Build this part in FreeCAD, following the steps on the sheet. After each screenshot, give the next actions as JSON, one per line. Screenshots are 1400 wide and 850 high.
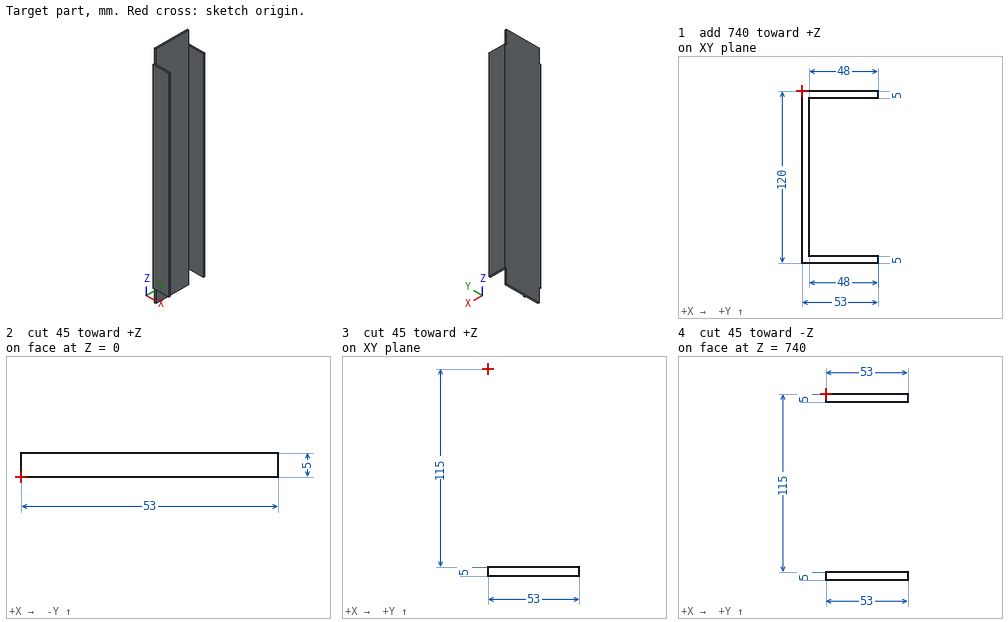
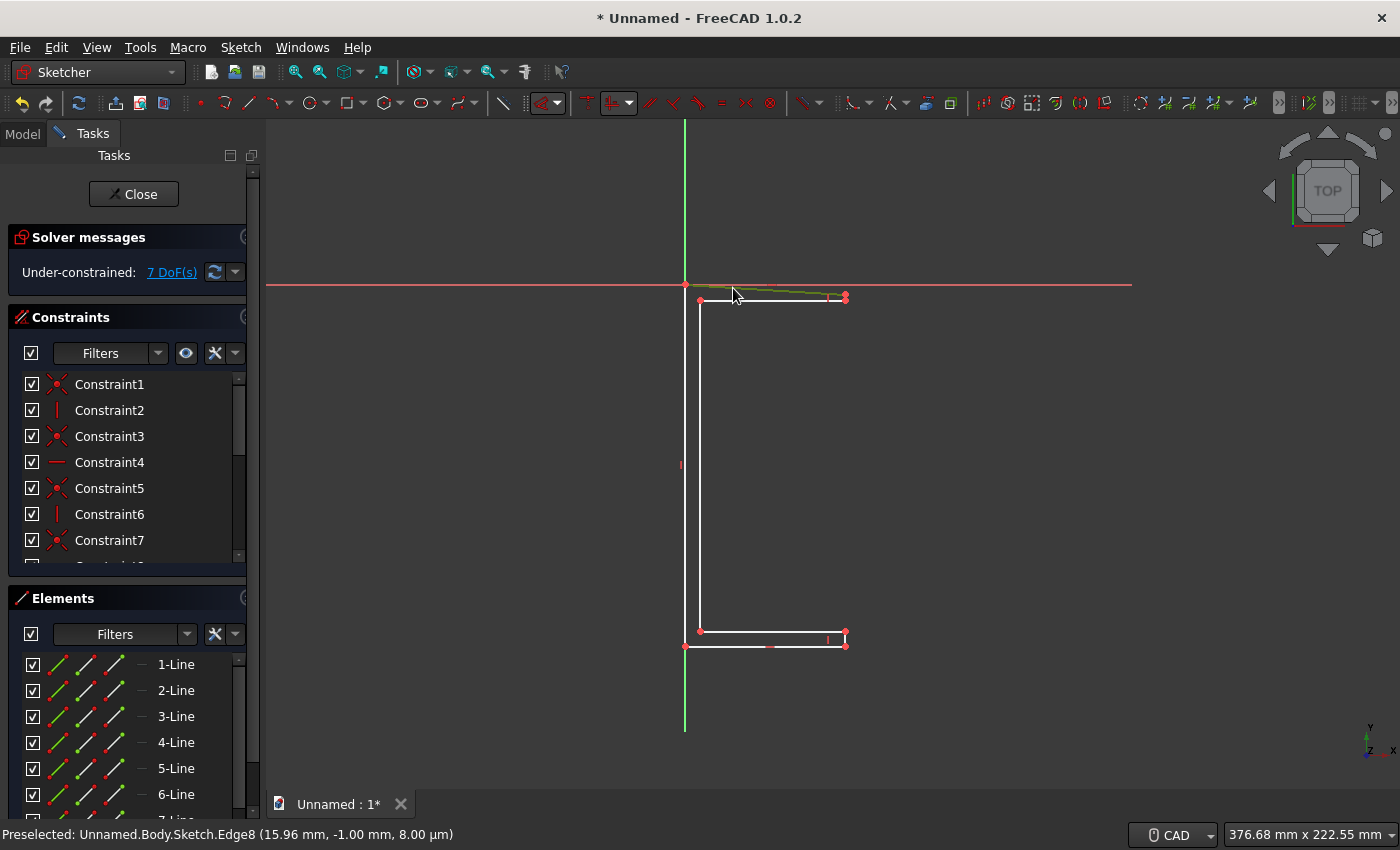
{"action": "left_click", "coordinate": [632, 104]}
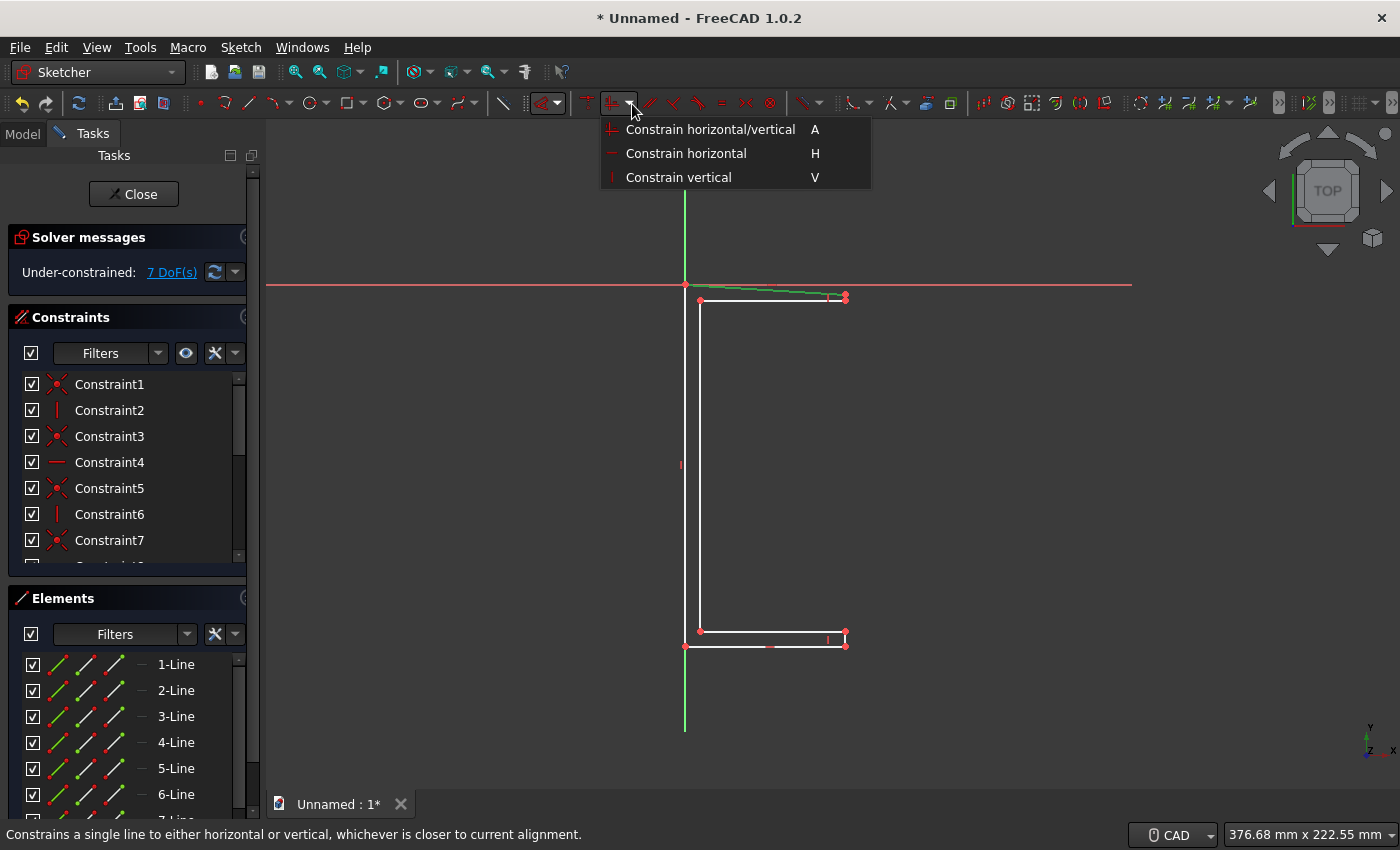
{"action": "left_click", "coordinate": [736, 153]}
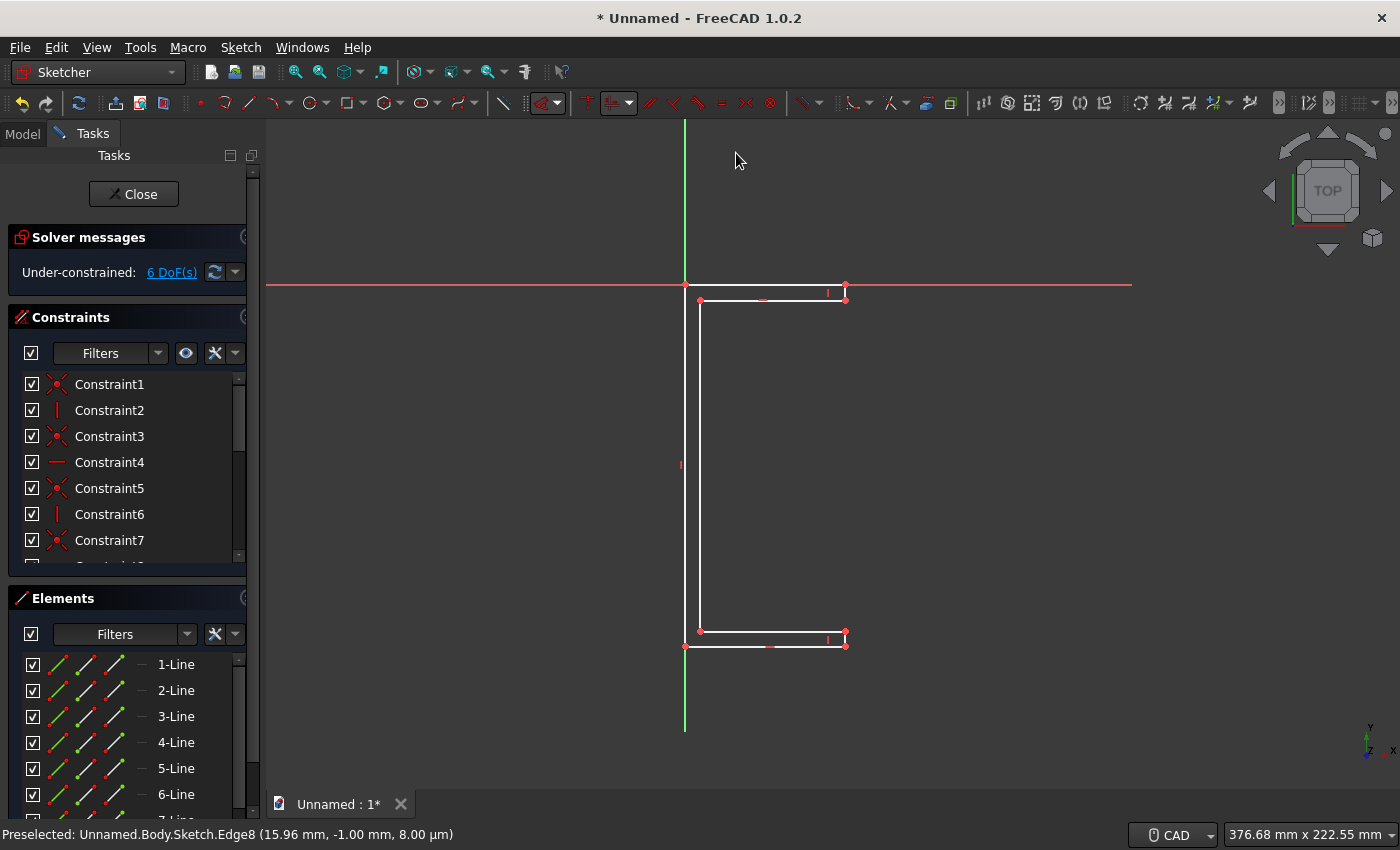
{"action": "scroll", "coordinate": [845, 640], "scroll_direction": "up", "scroll_amount": 5}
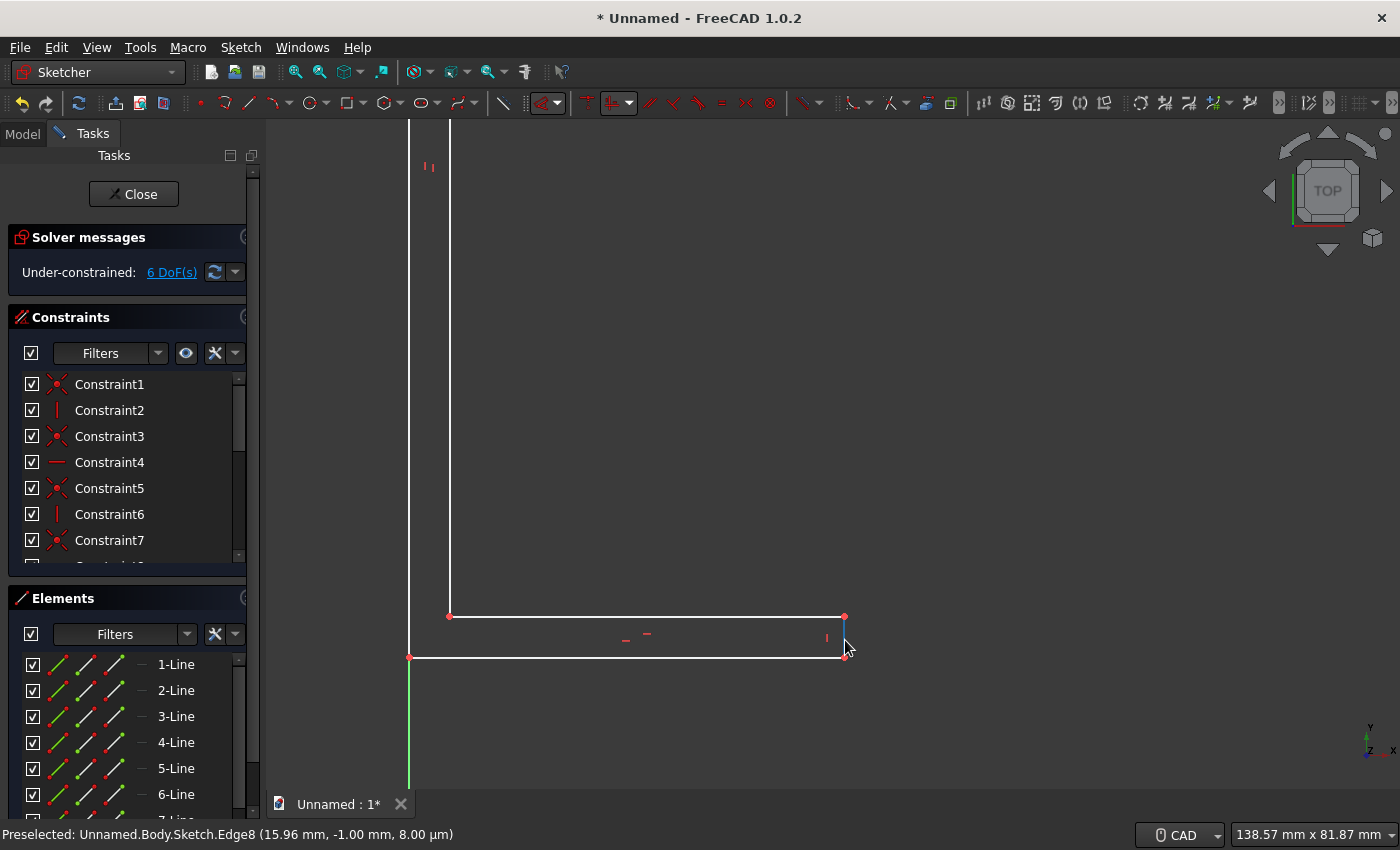
{"action": "left_click", "coordinate": [844, 637]}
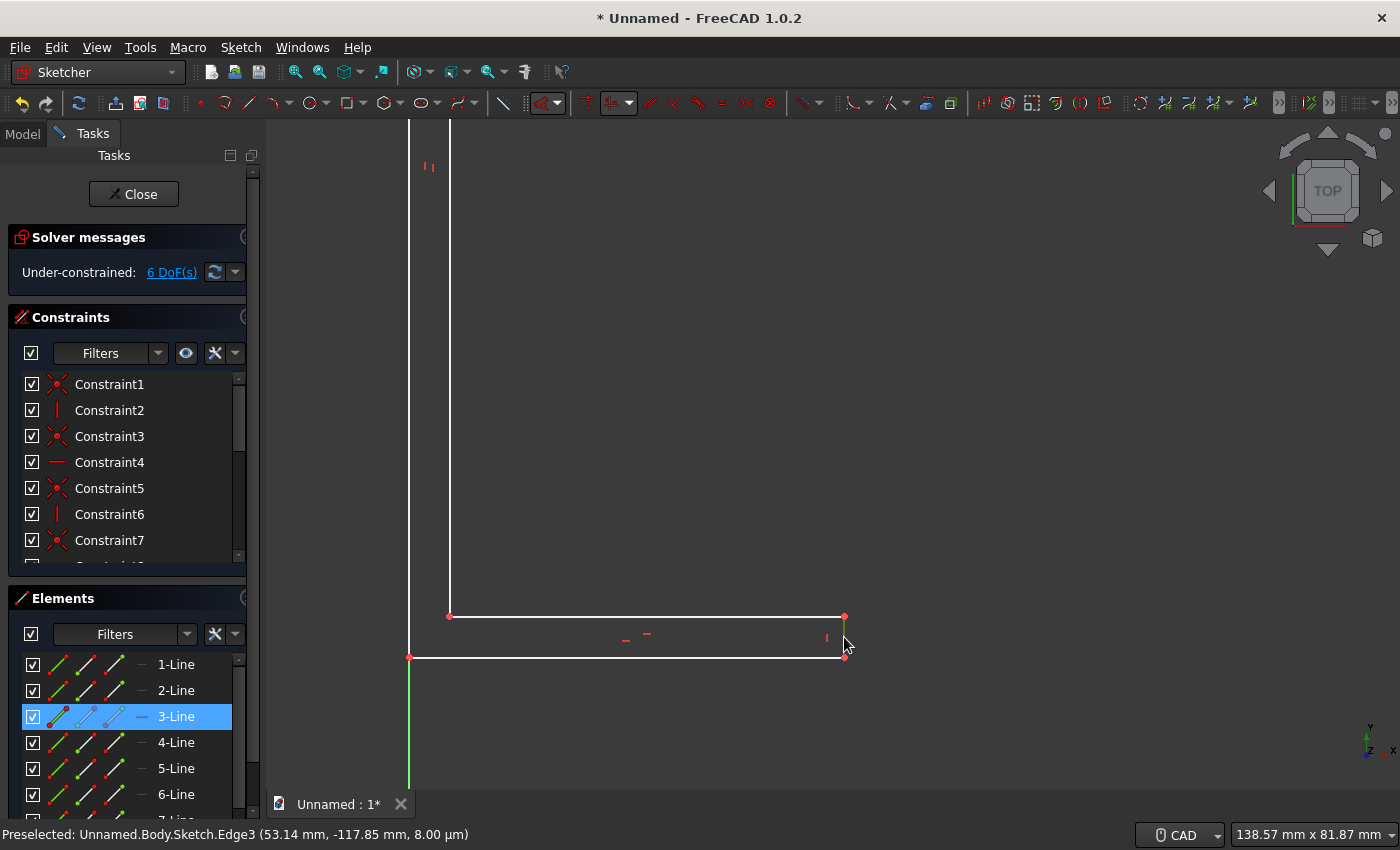
{"action": "key", "text": "i"}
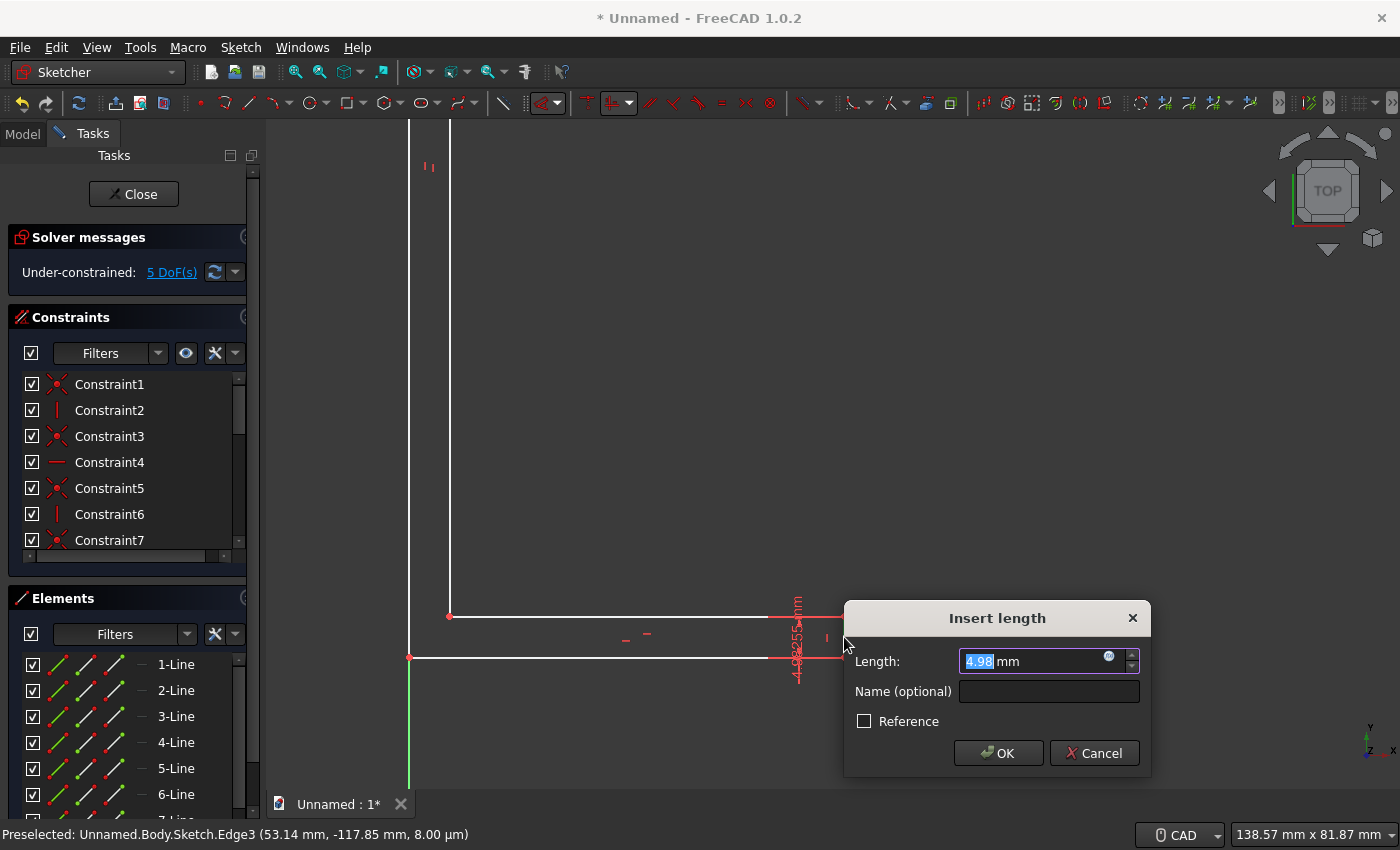
{"action": "type", "text": "5"}
{"action": "key", "text": "Return"}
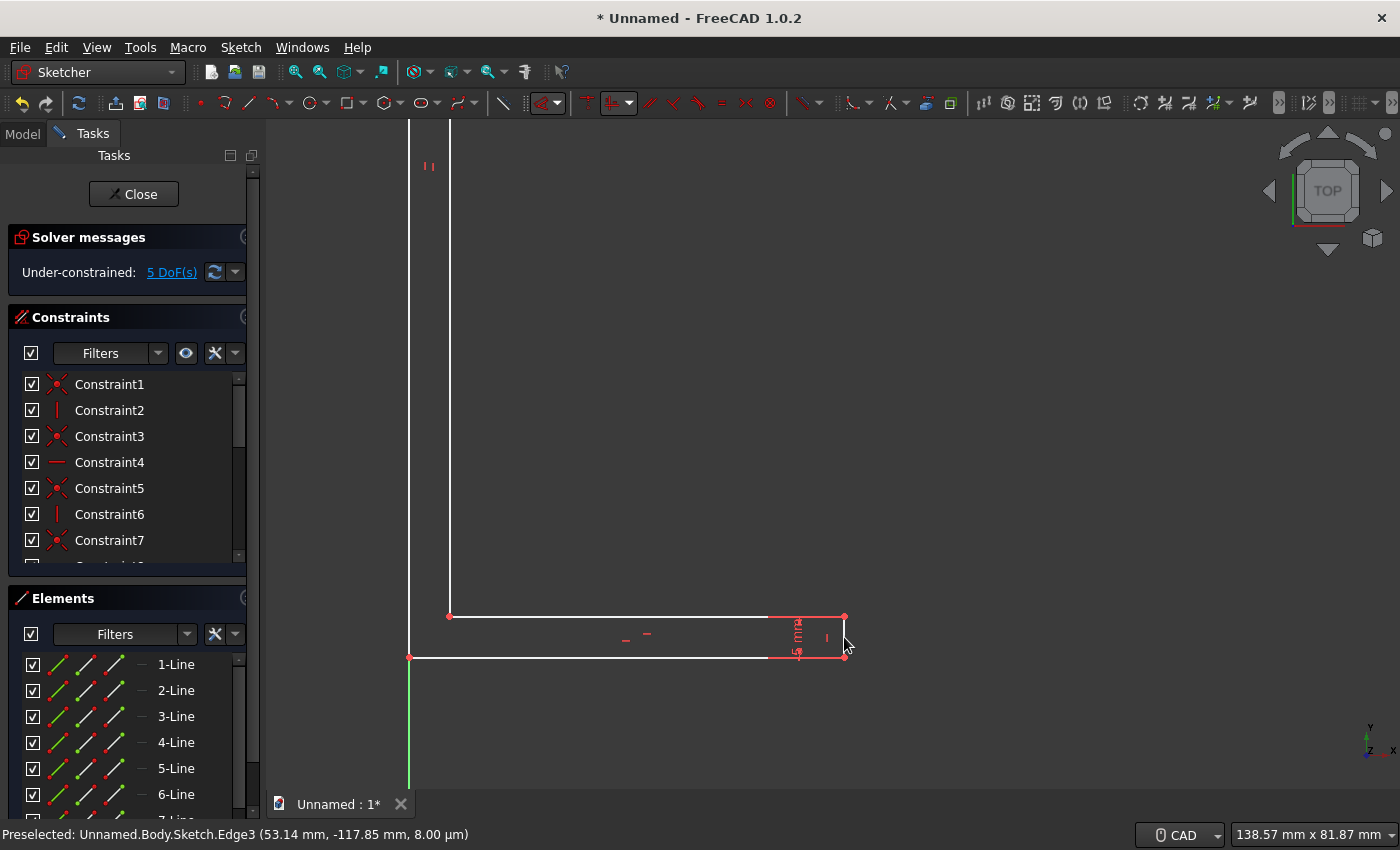
{"action": "scroll", "coordinate": [877, 690], "scroll_direction": "down", "scroll_amount": 4}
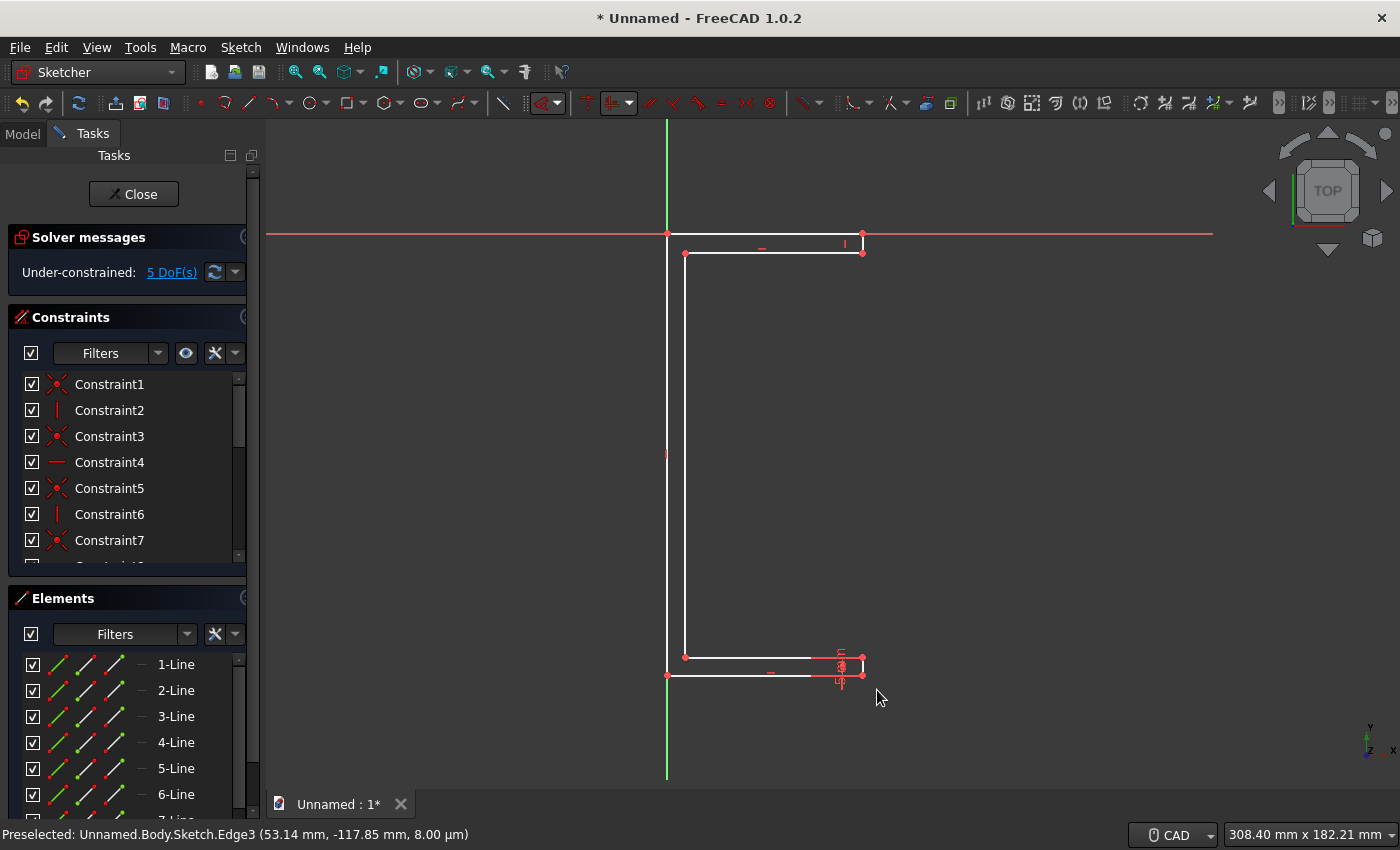
{"action": "scroll", "coordinate": [863, 247], "scroll_direction": "up", "scroll_amount": 5}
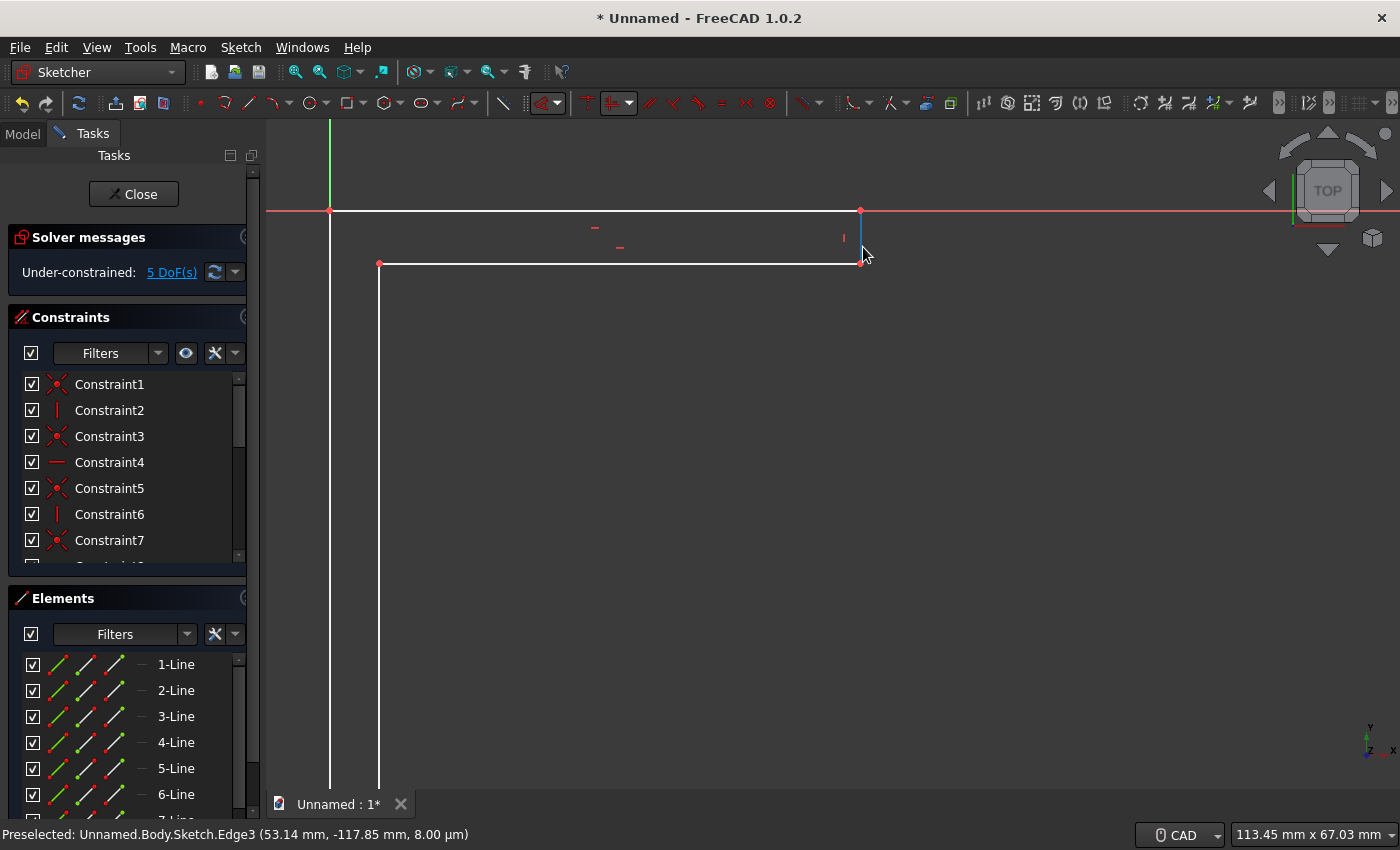
{"action": "left_click", "coordinate": [861, 248]}